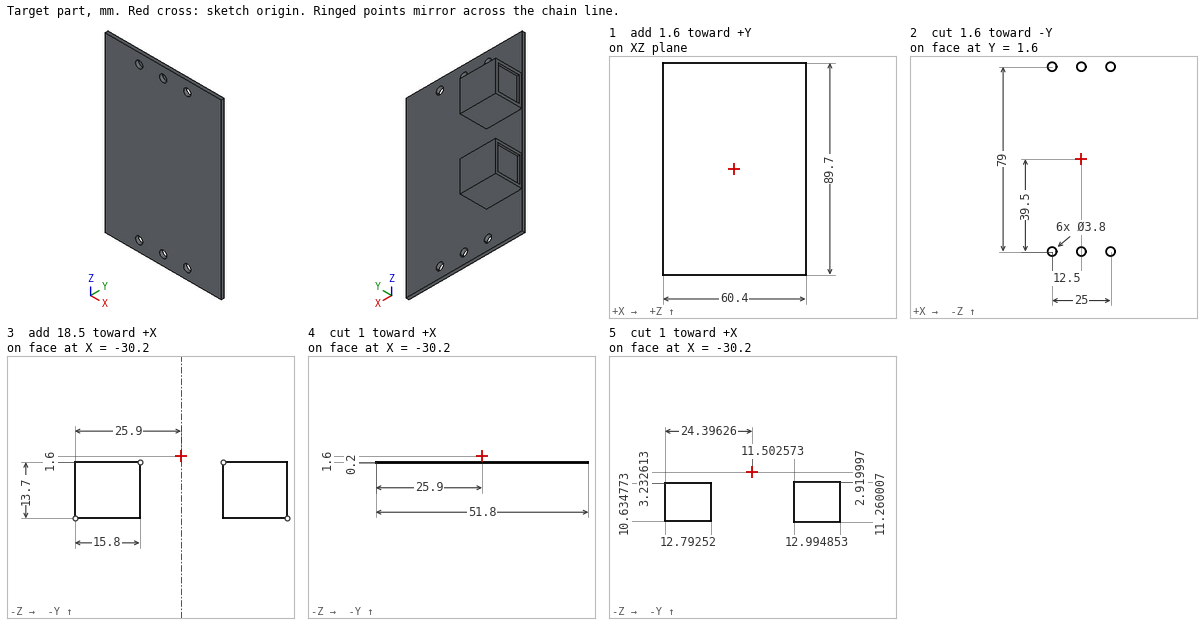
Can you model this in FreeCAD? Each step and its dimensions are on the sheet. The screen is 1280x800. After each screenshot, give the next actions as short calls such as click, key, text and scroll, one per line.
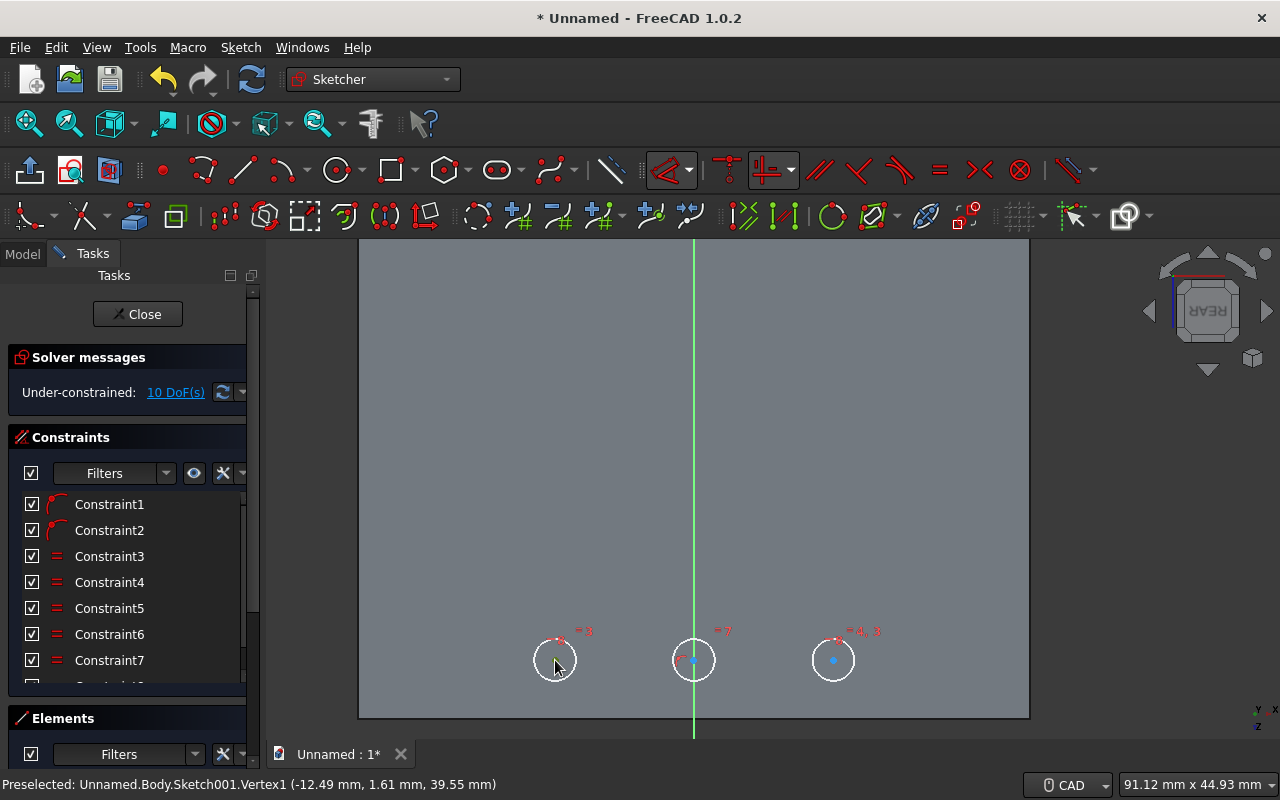
scroll(711, 646, down, 5)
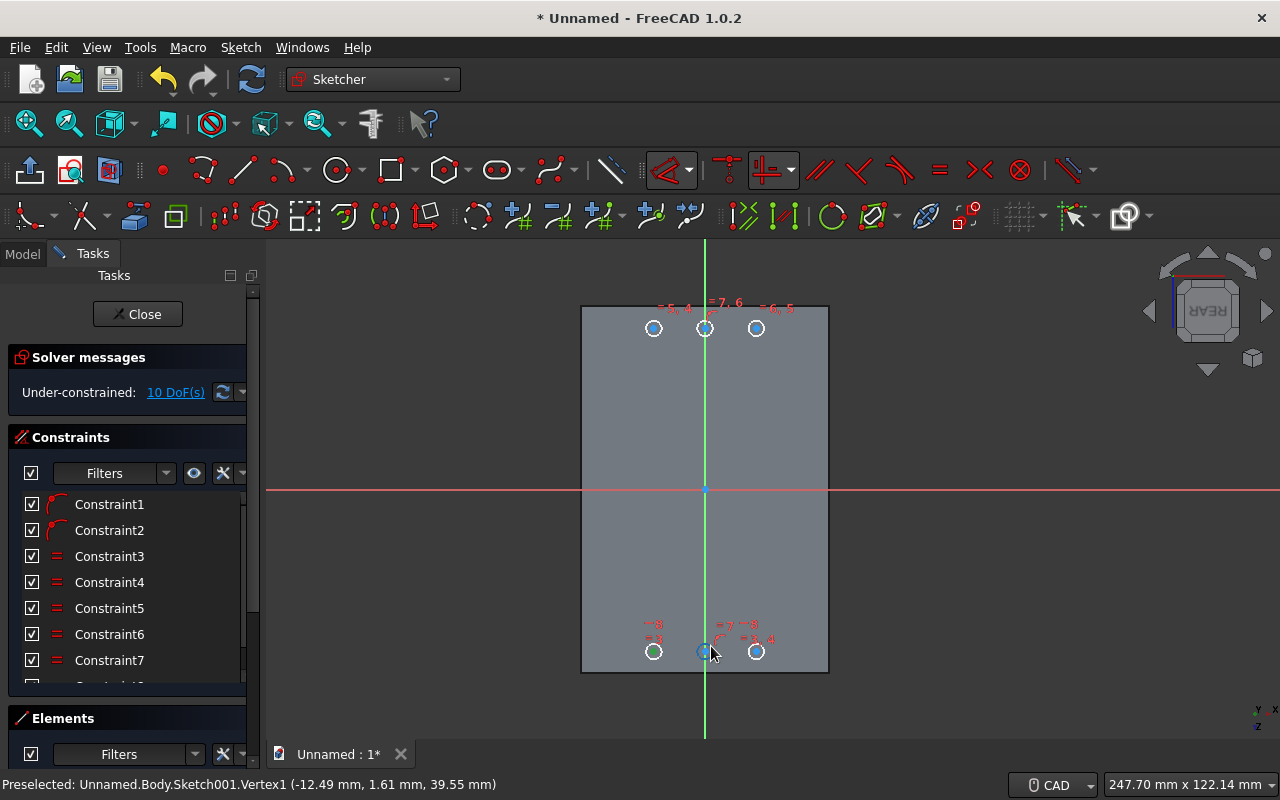
click(654, 328)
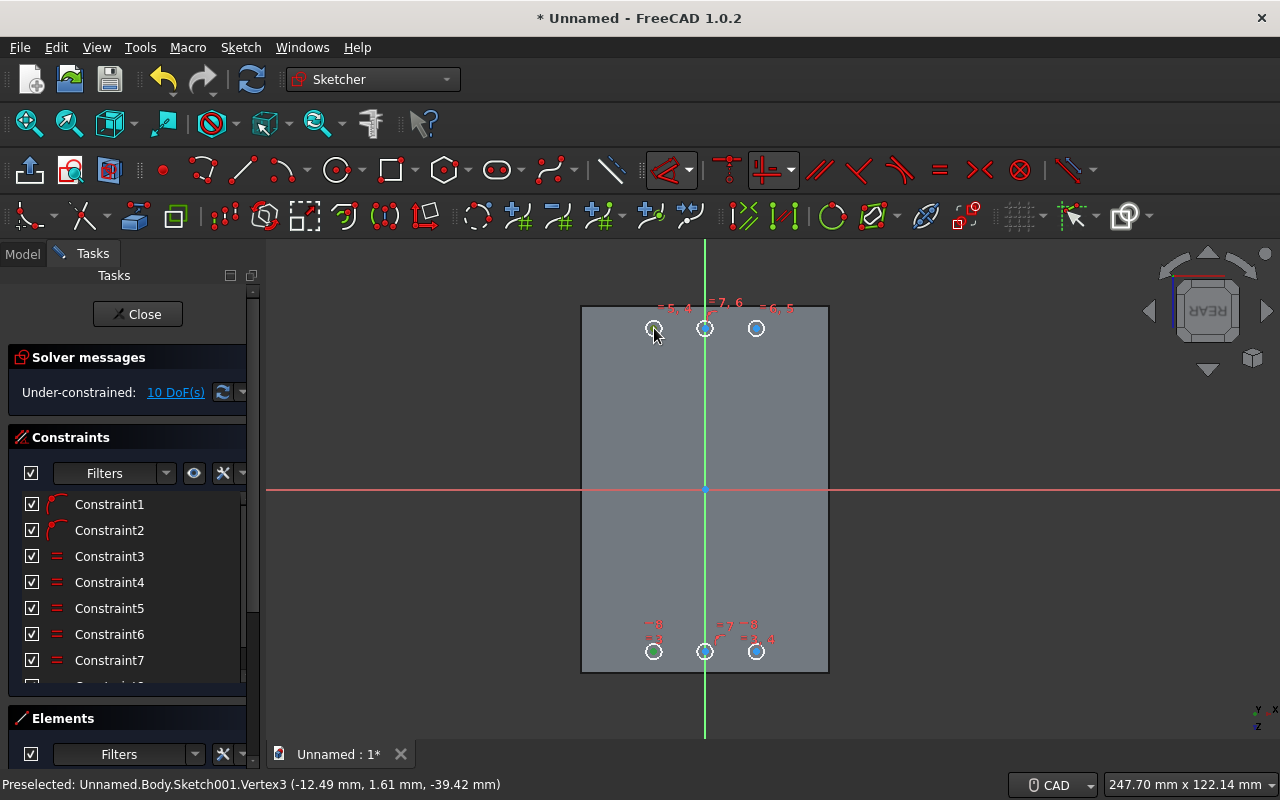
key(v)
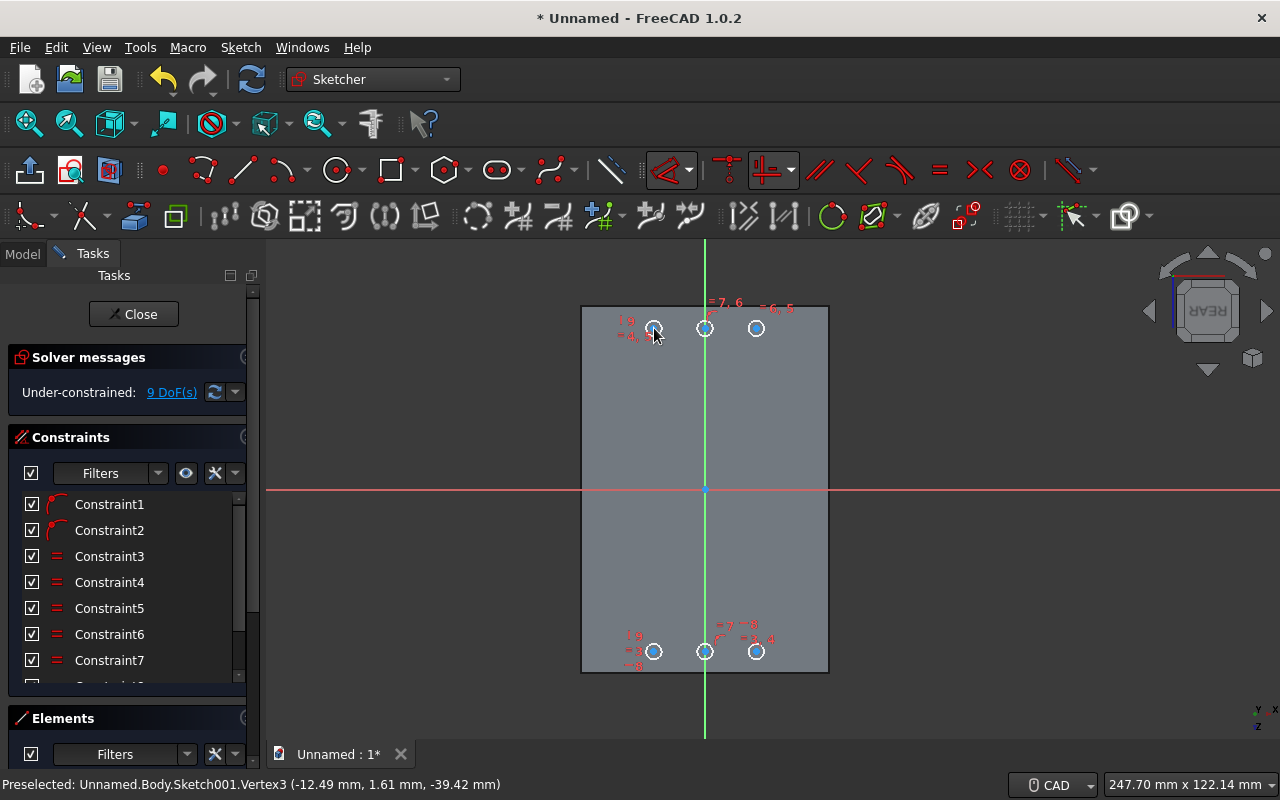
click(756, 652)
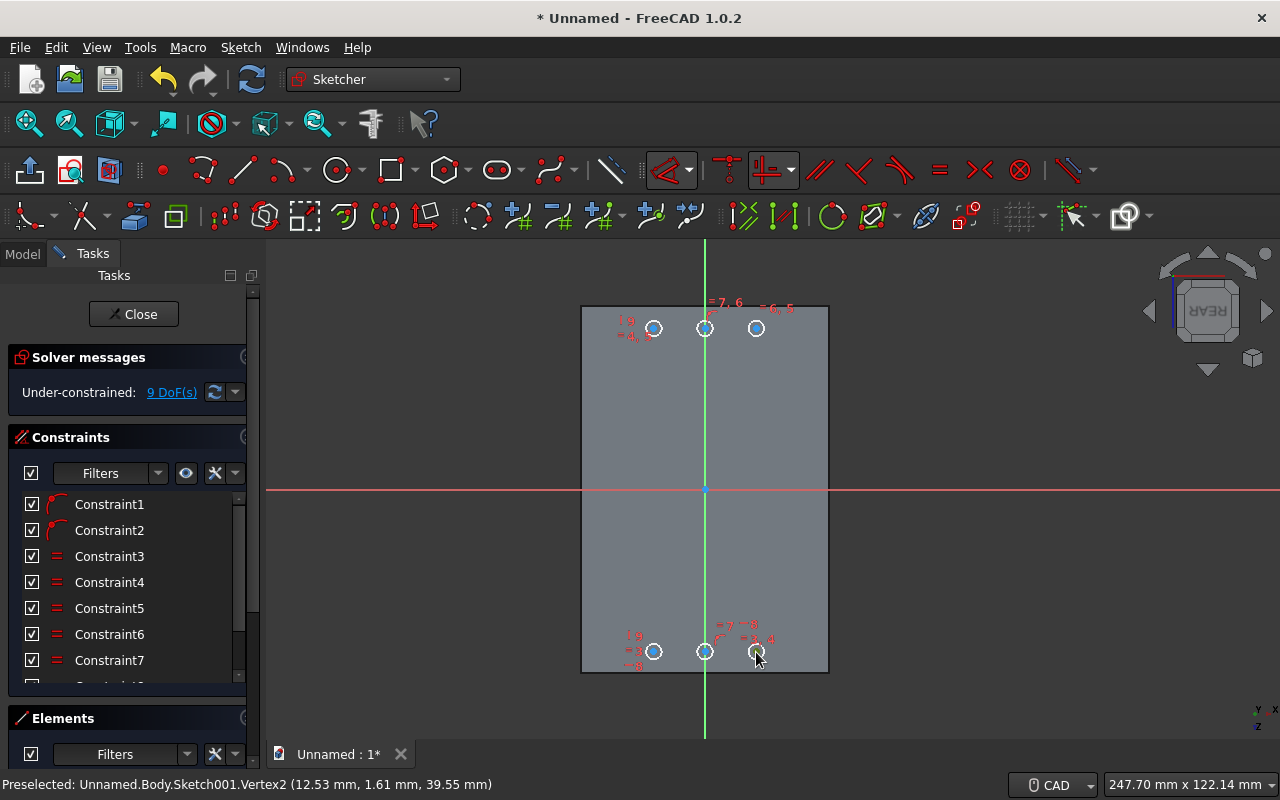
click(756, 328)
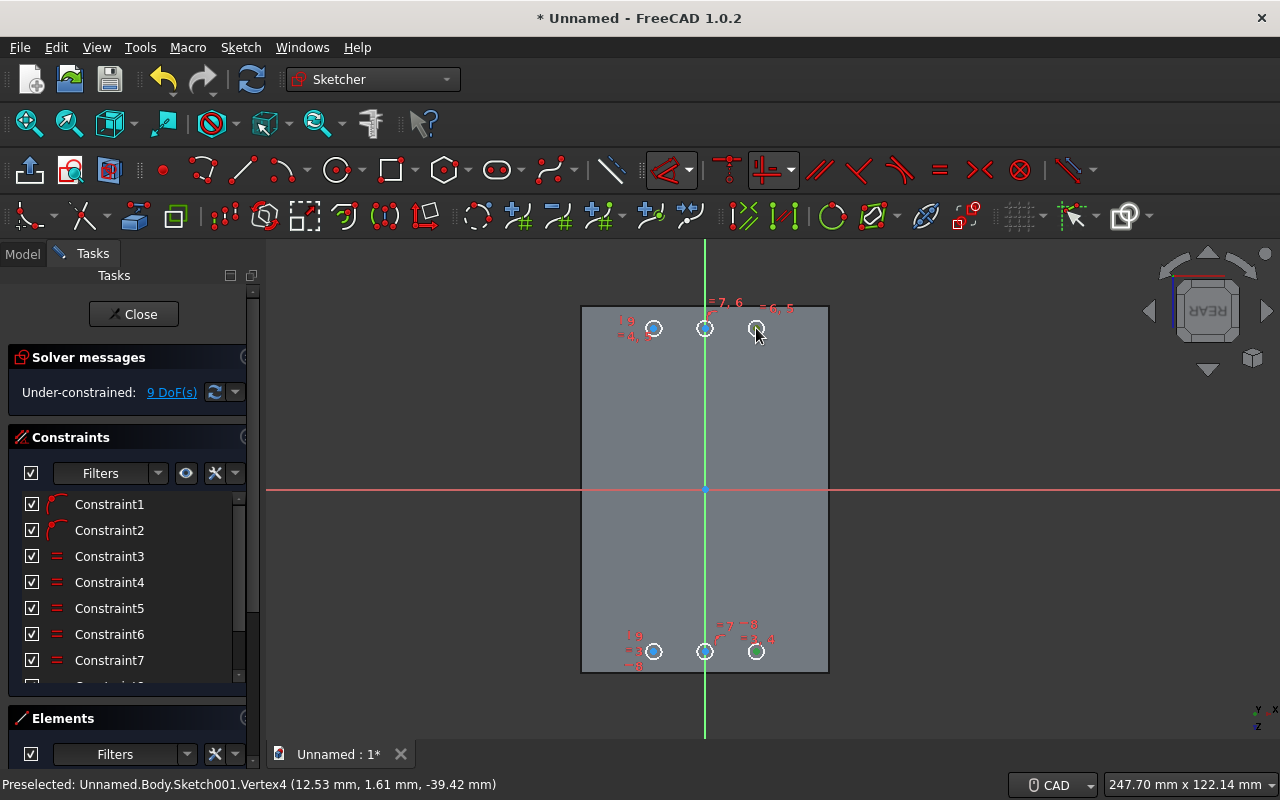
key(v)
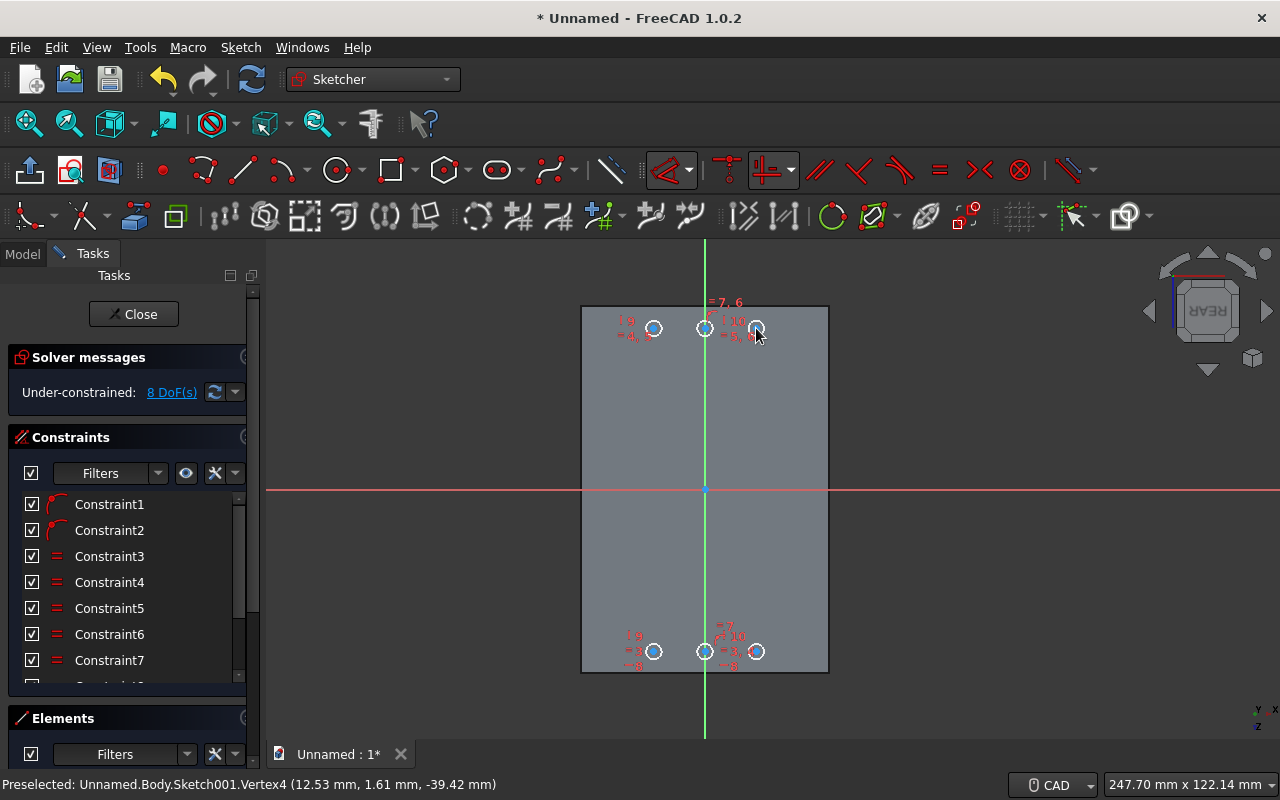
click(654, 328)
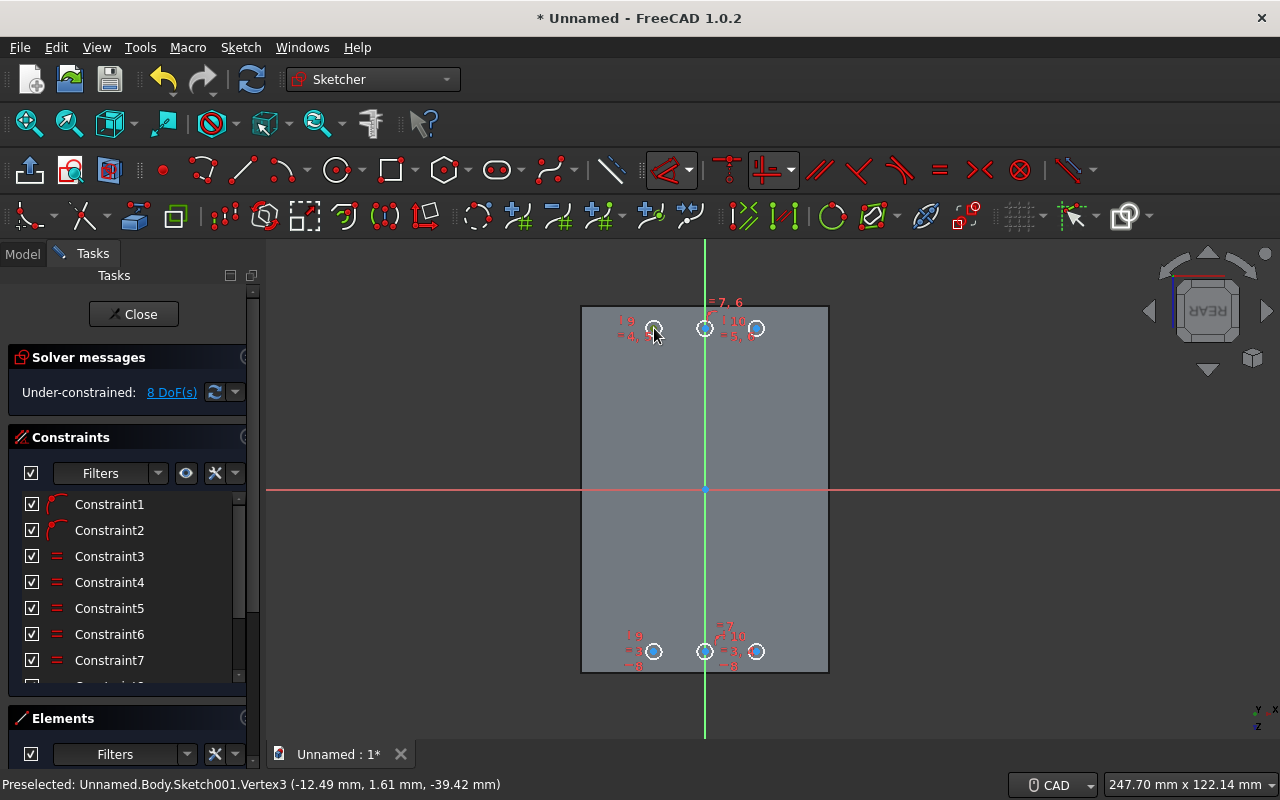
click(756, 328)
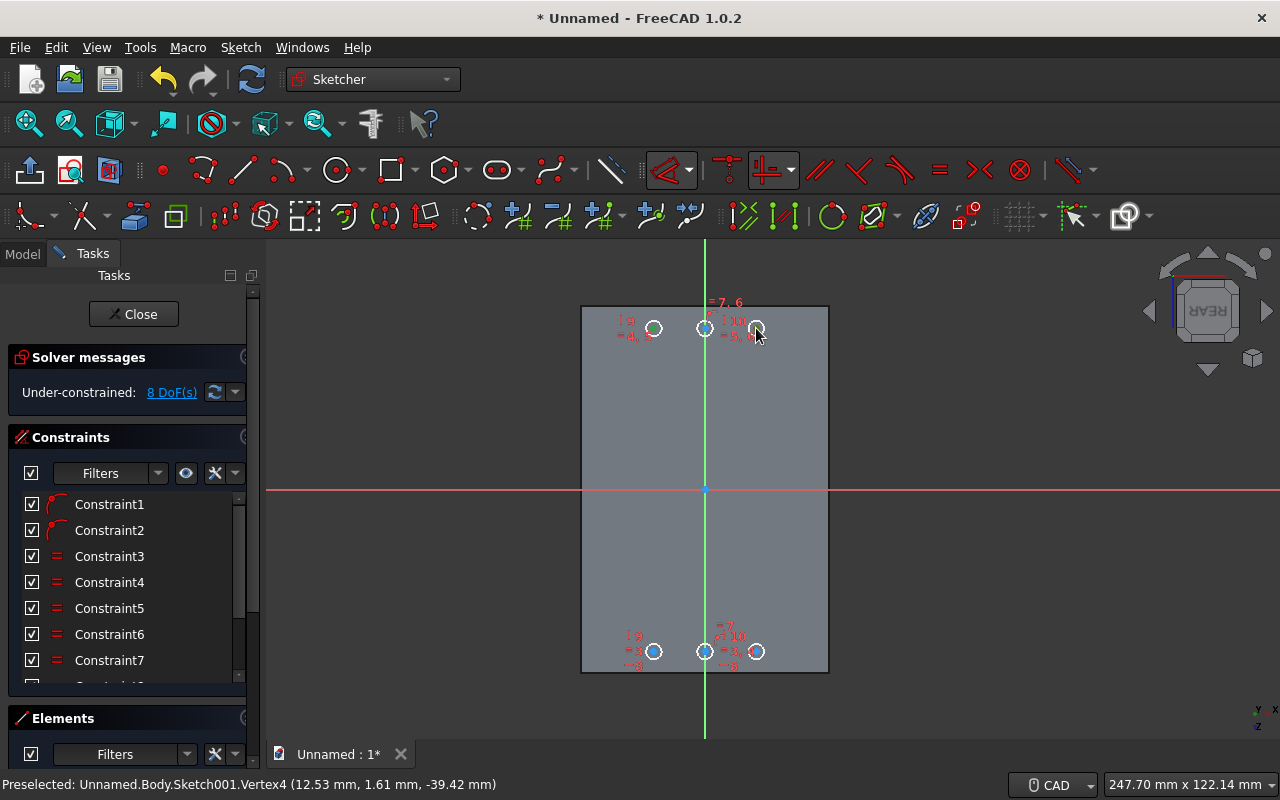
click(794, 170)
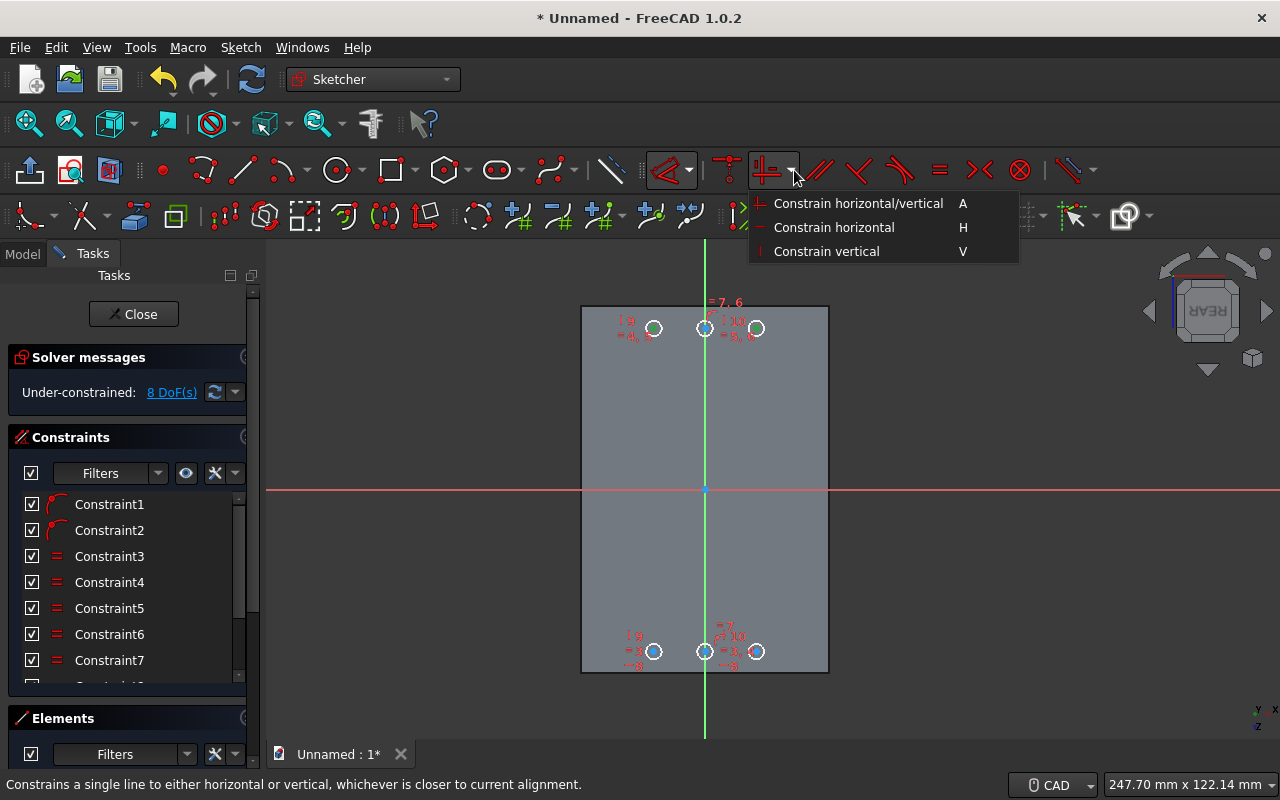
click(884, 227)